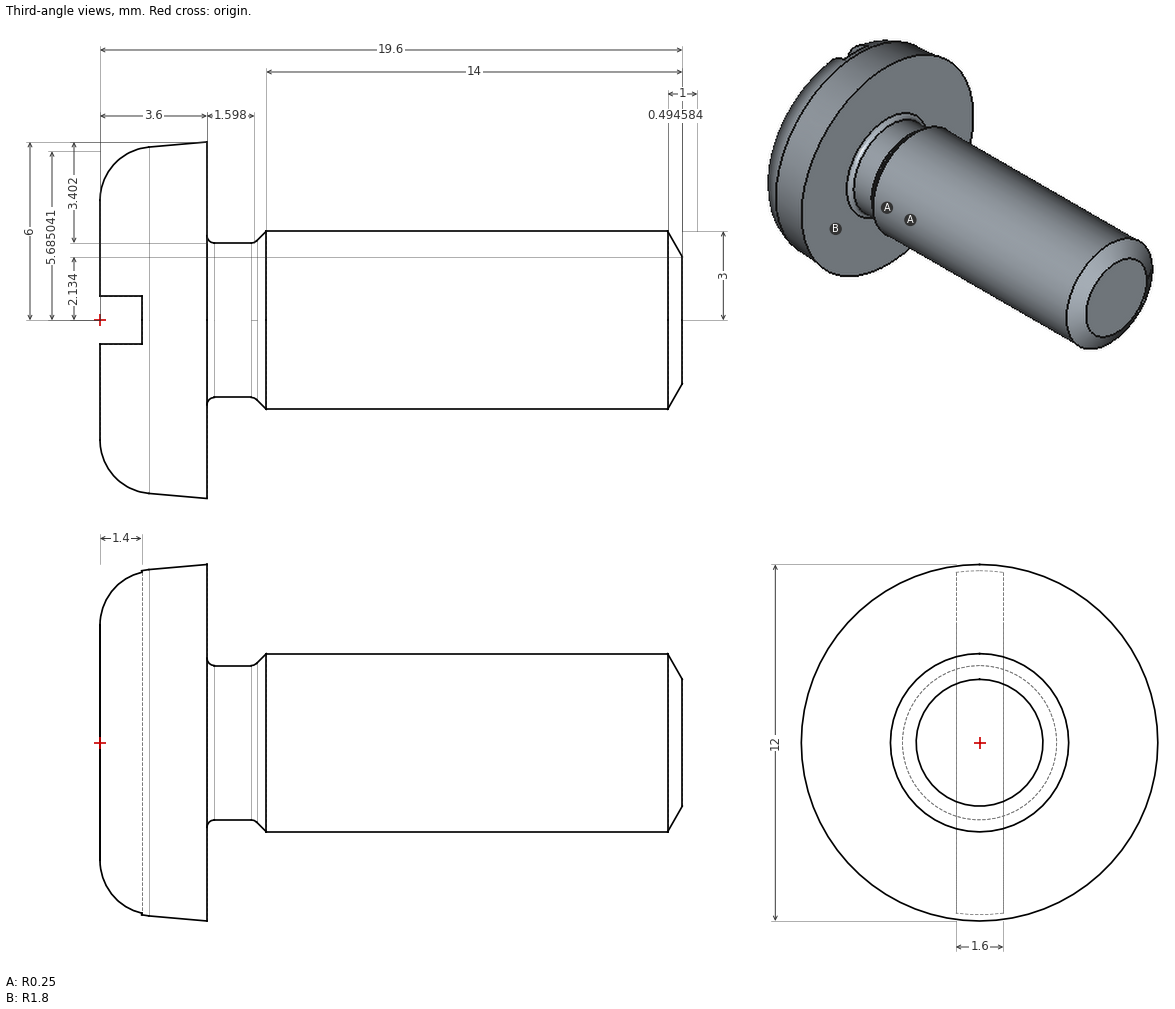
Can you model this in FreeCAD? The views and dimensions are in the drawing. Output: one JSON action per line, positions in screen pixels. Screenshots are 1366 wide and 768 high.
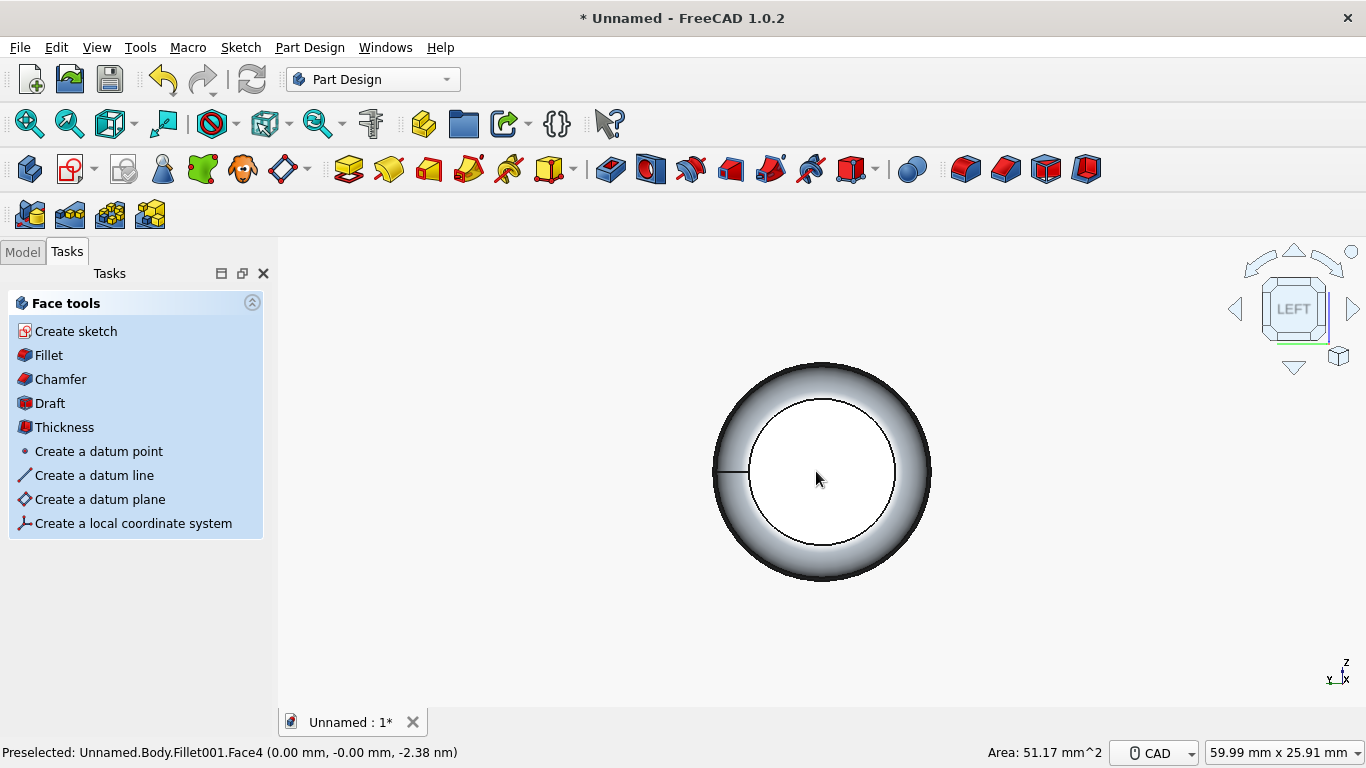
{"action": "left_click", "coordinate": [70, 170]}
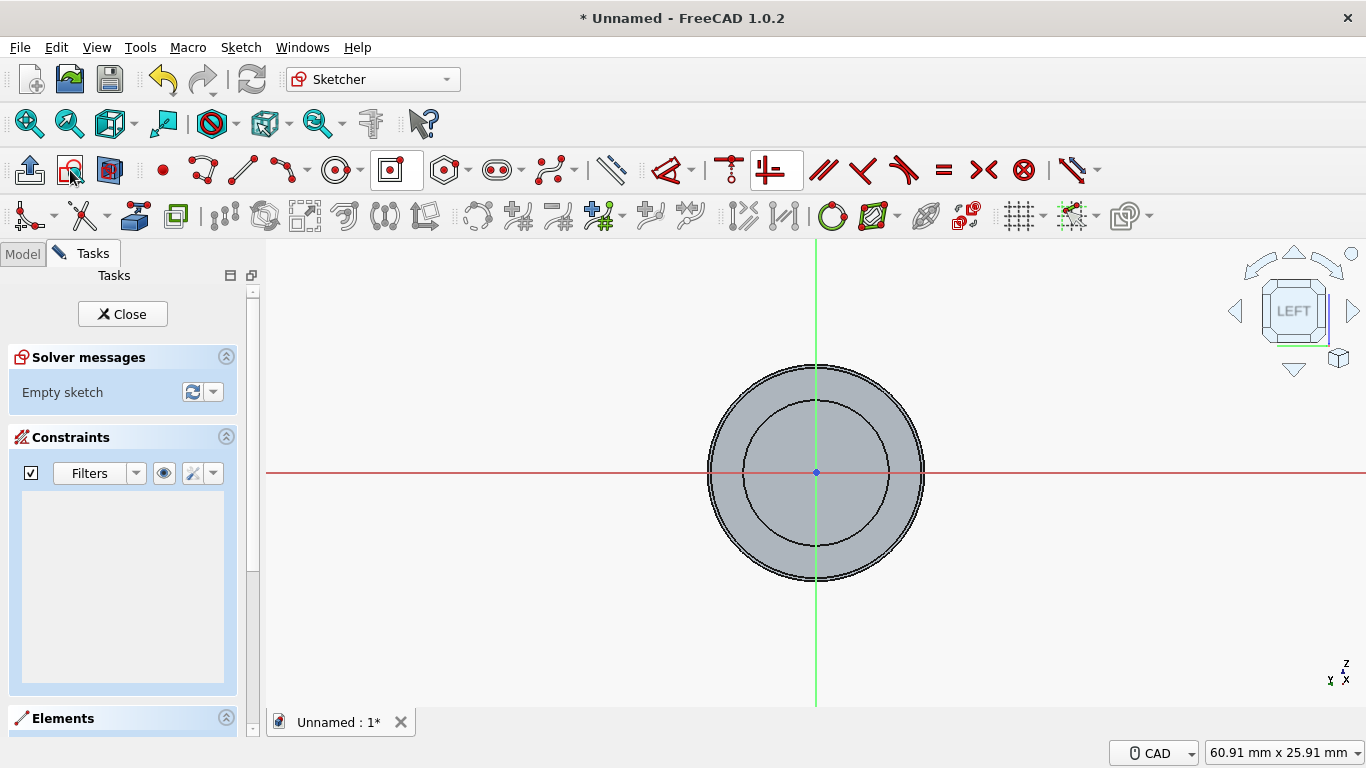
{"action": "left_click", "coordinate": [390, 170]}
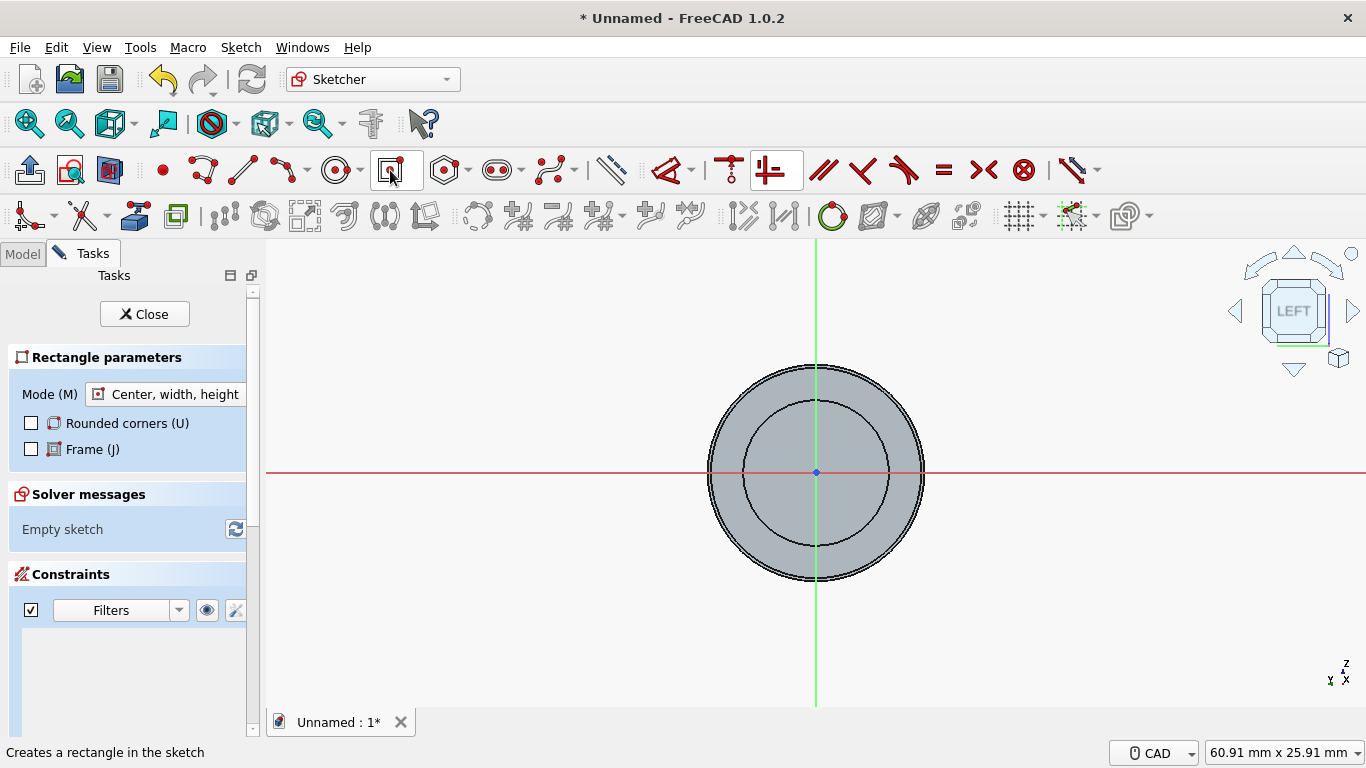
{"action": "left_click", "coordinate": [816, 473]}
{"action": "mouse_move", "coordinate": [830, 365]}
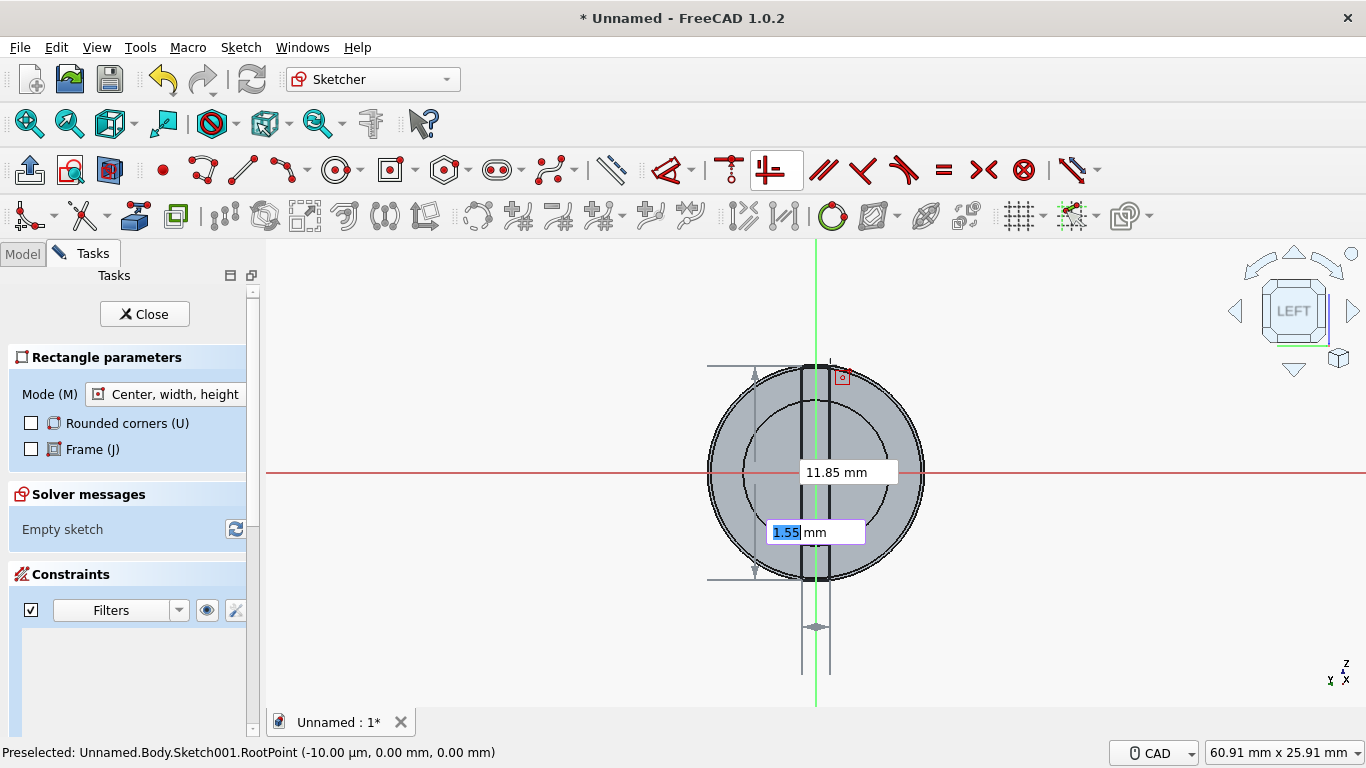
{"action": "type", "text": "1.6"}
{"action": "key", "text": "Tab"}
{"action": "type", "text": "12"}
{"action": "key", "text": "Return"}
{"action": "key", "text": "Escape"}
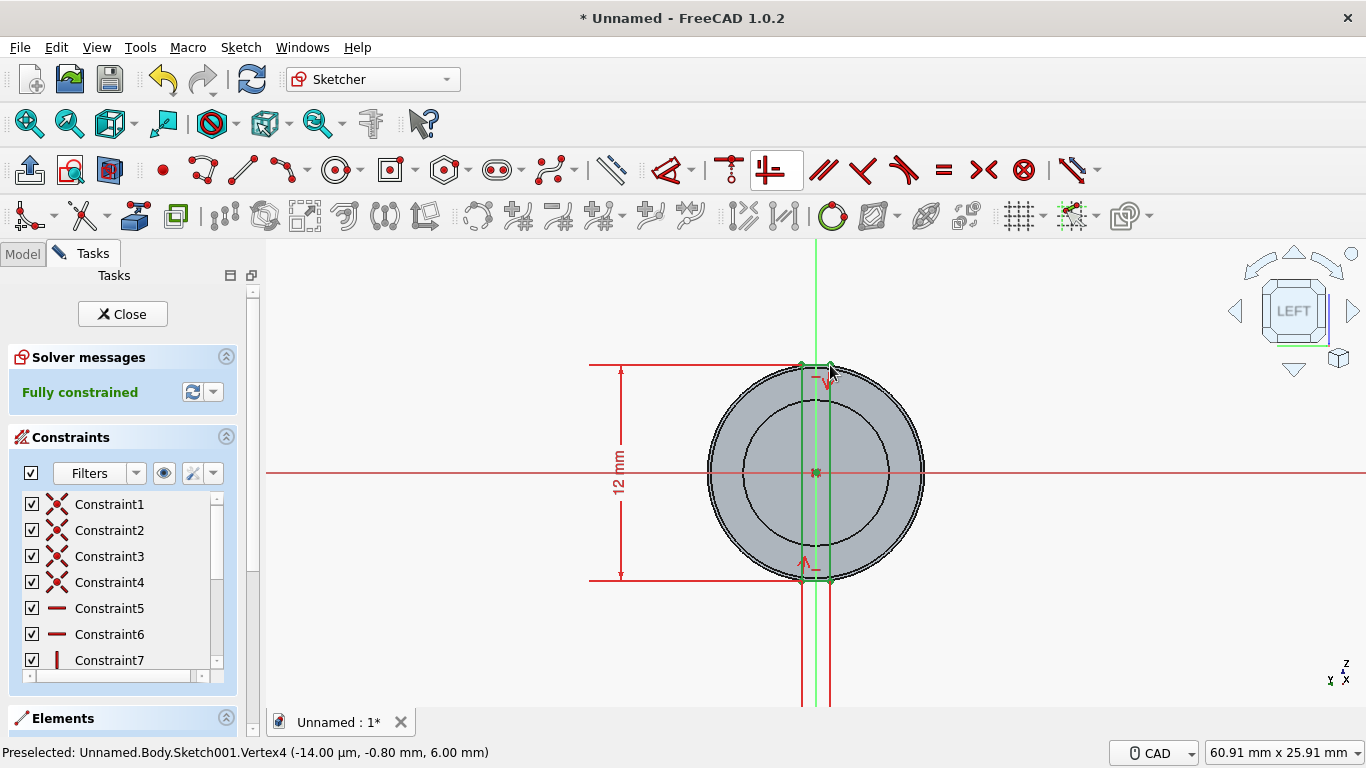
{"action": "left_click", "coordinate": [123, 314]}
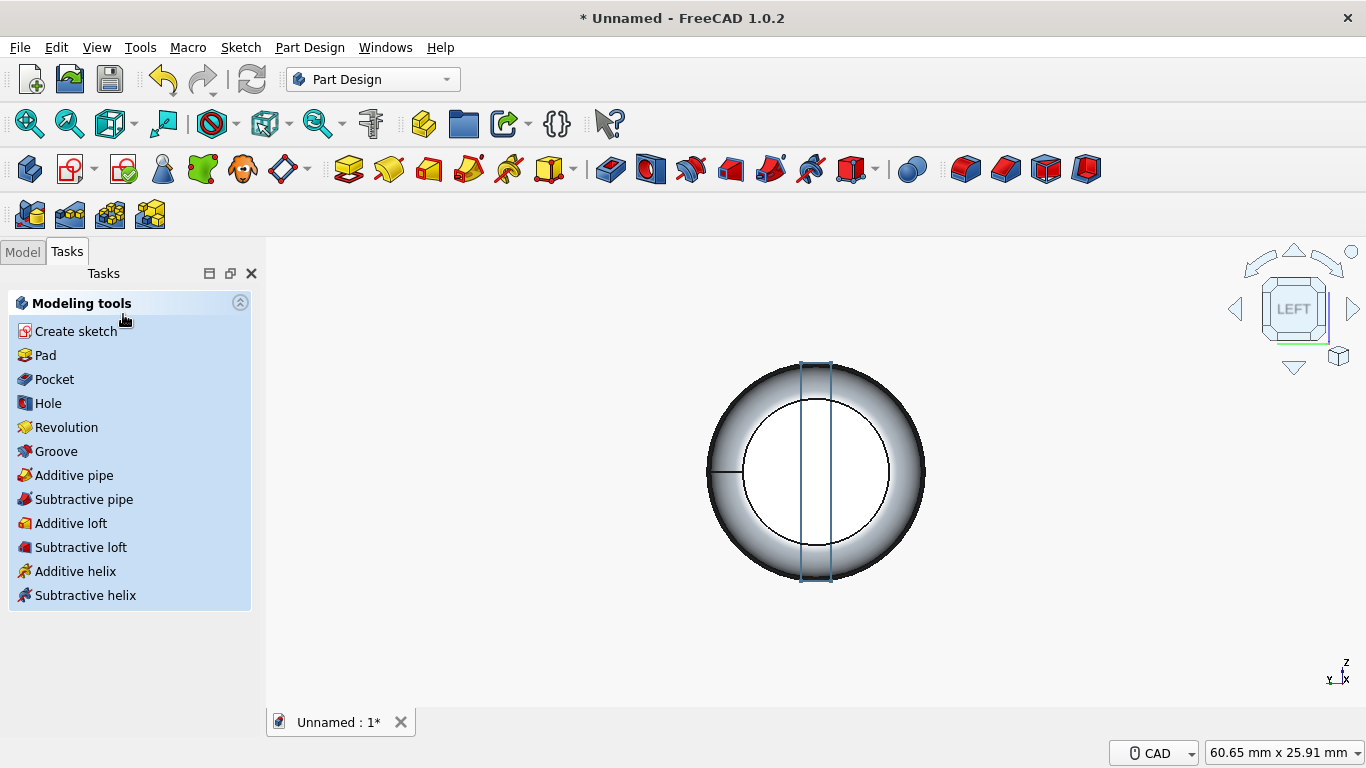
{"action": "left_click", "coordinate": [612, 170]}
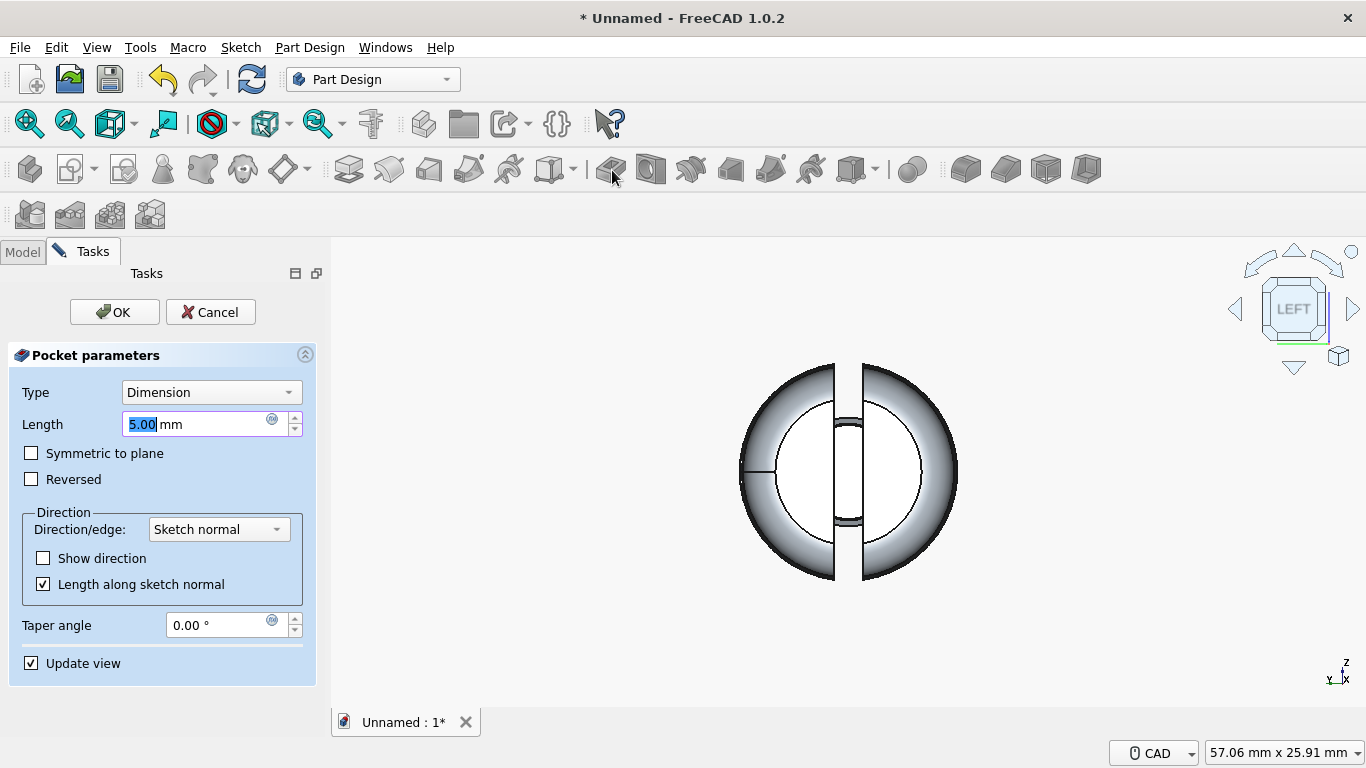
{"action": "type", "text": "1.4"}
{"action": "key", "text": "Tab"}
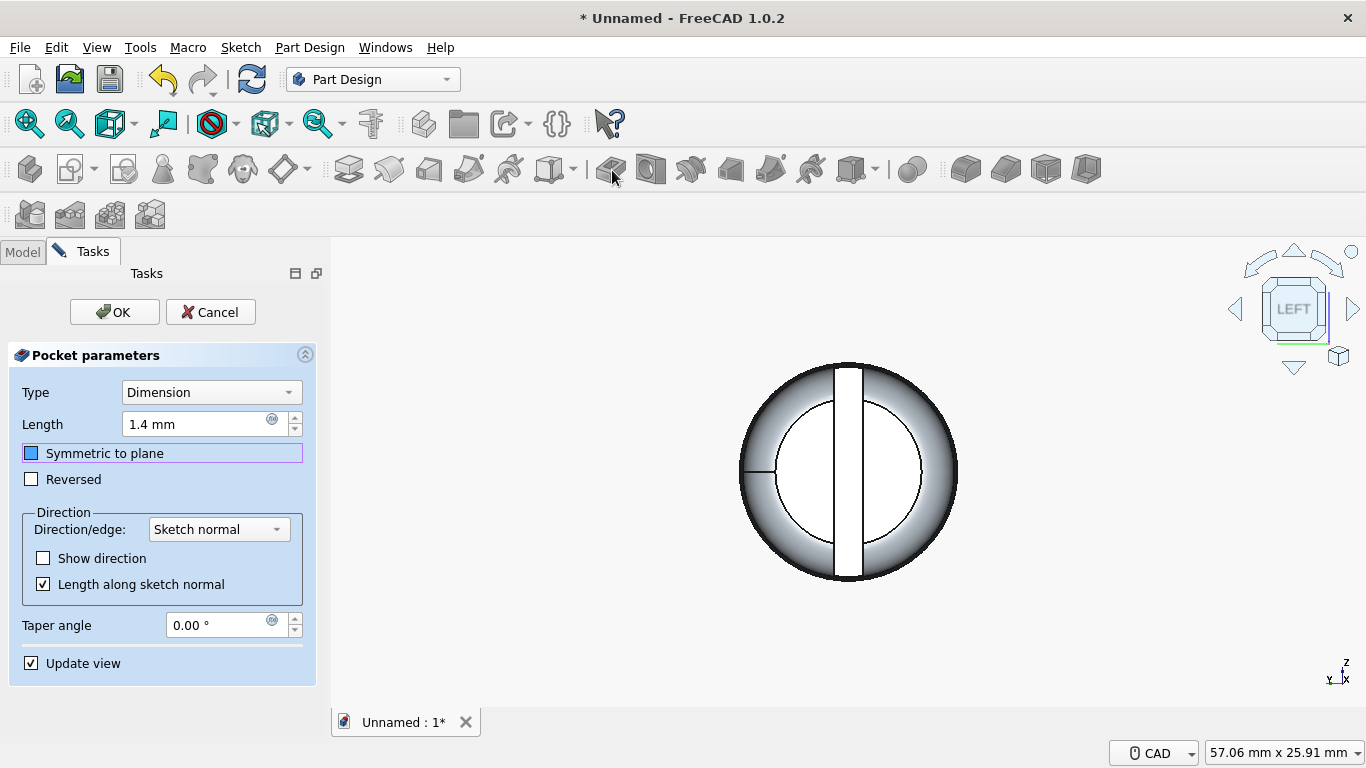
{"action": "left_click", "coordinate": [115, 312]}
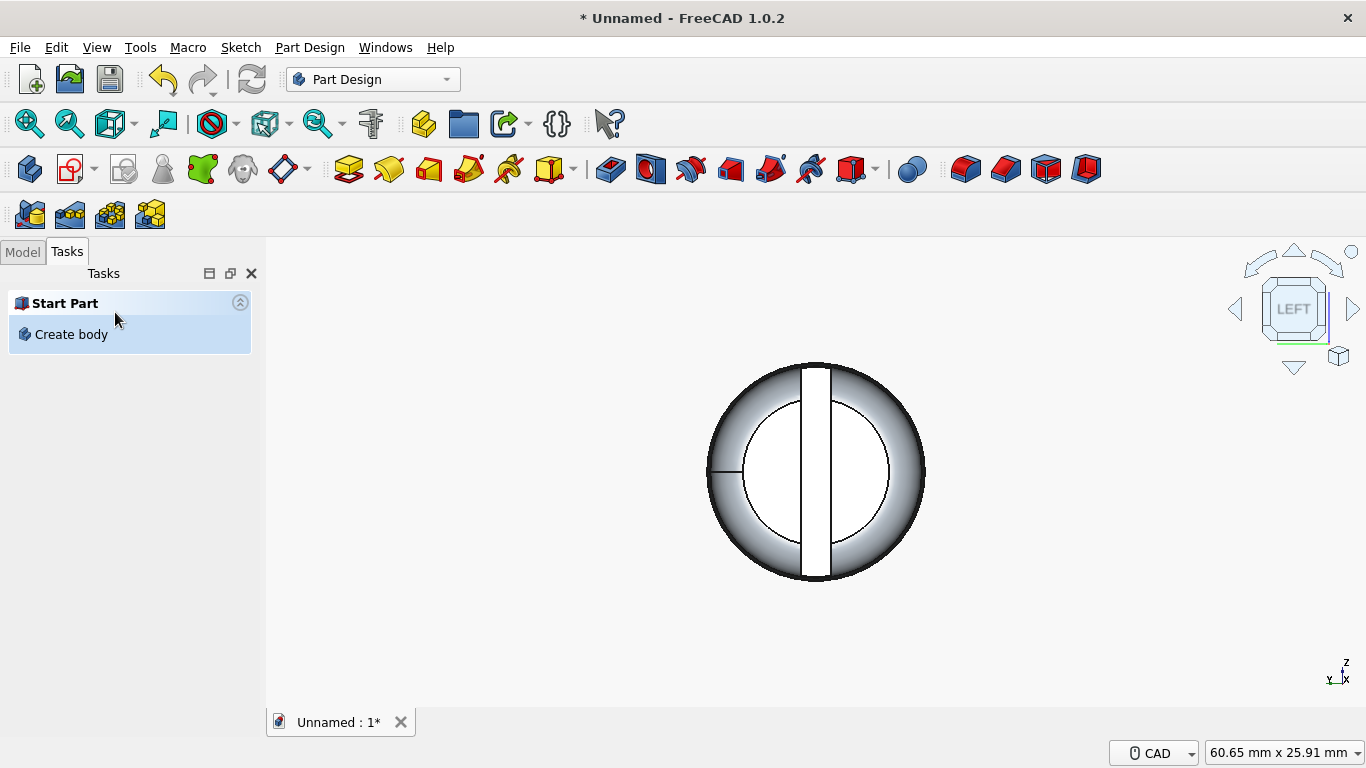
{"action": "left_click", "coordinate": [70, 170]}